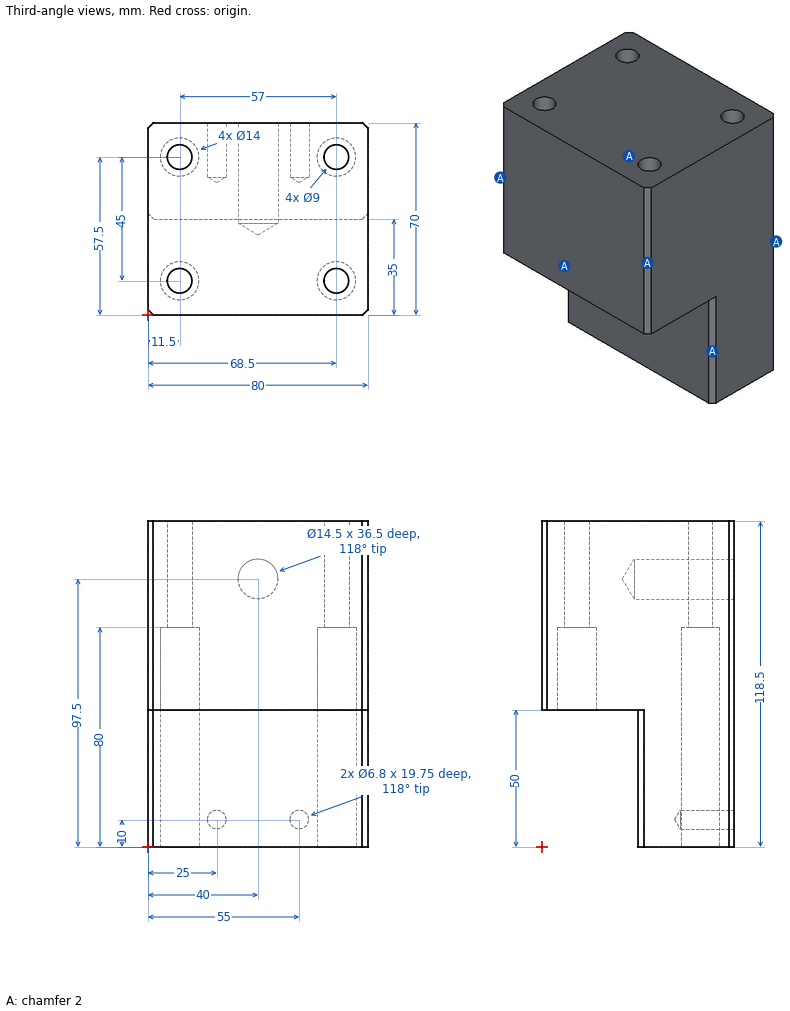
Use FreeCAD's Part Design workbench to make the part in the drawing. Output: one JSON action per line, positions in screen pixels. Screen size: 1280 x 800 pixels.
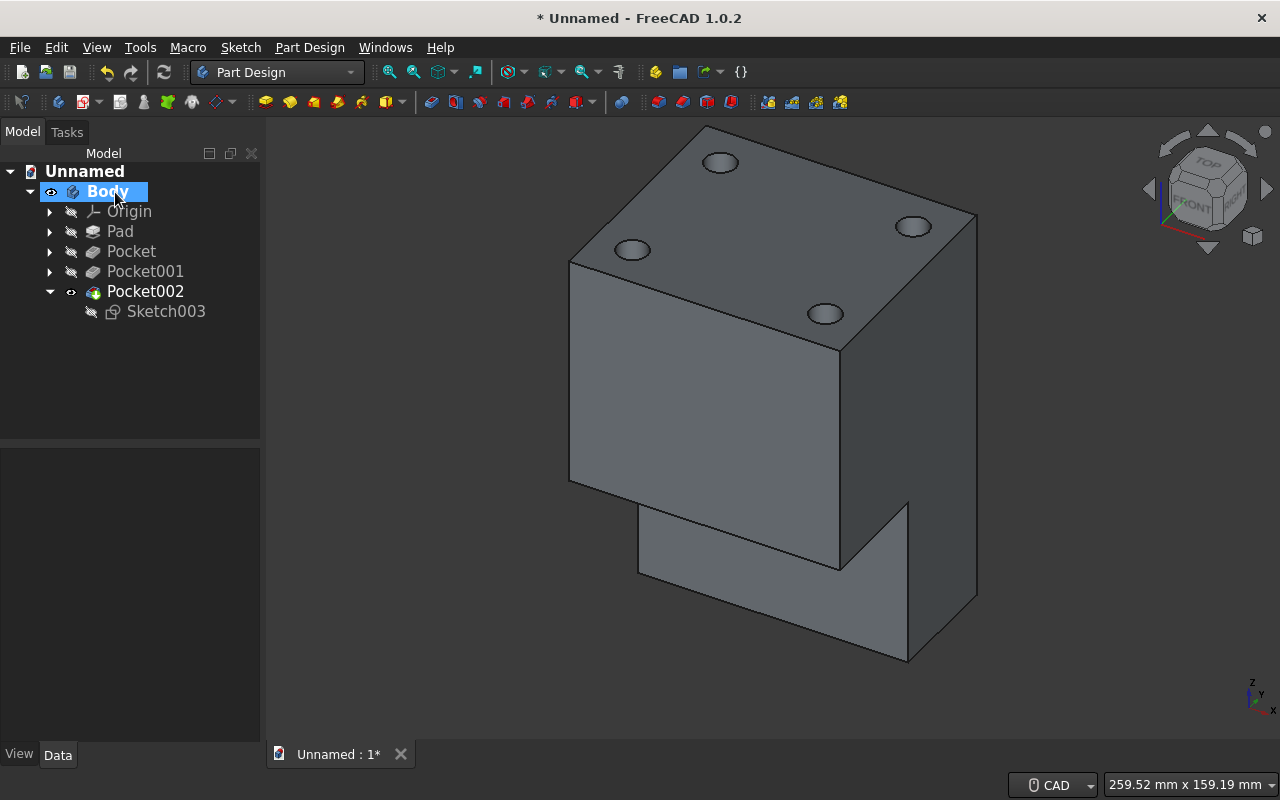
{"action": "key", "text": "4"}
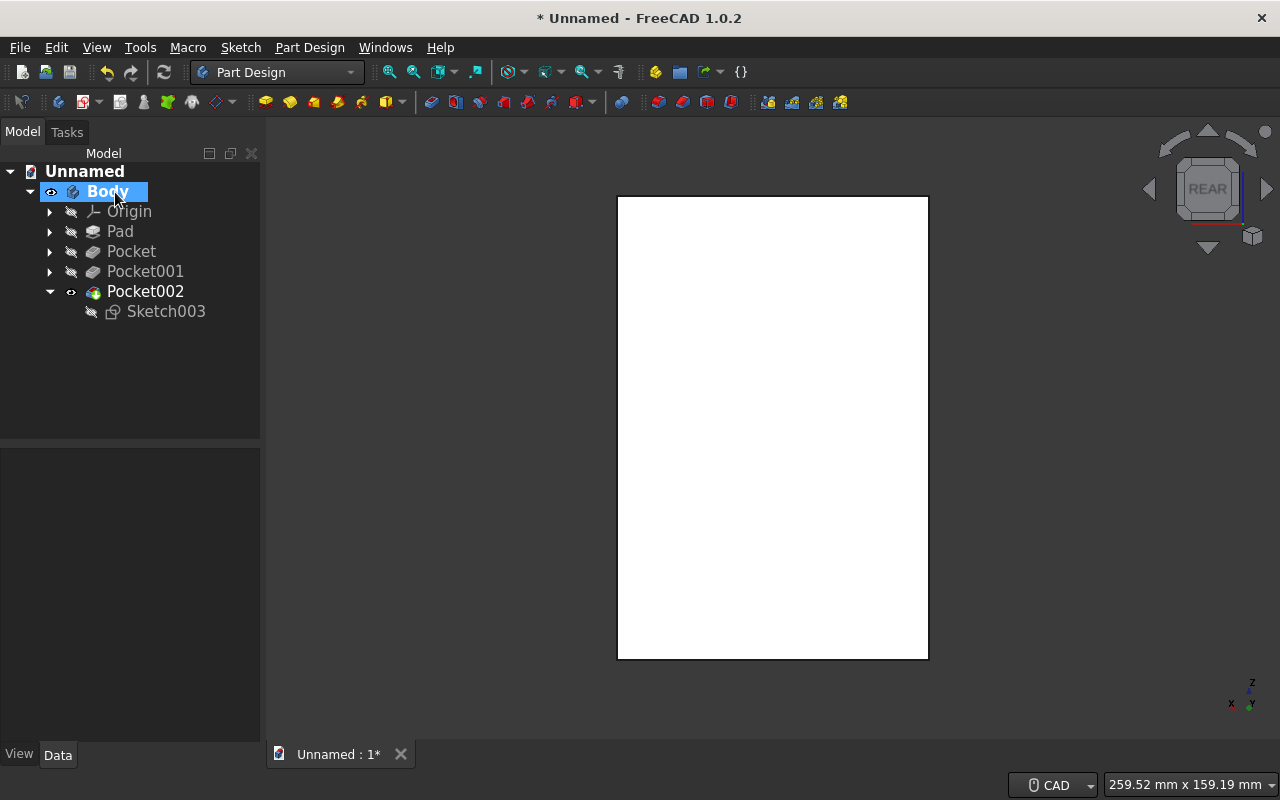
{"action": "left_click", "coordinate": [773, 361]}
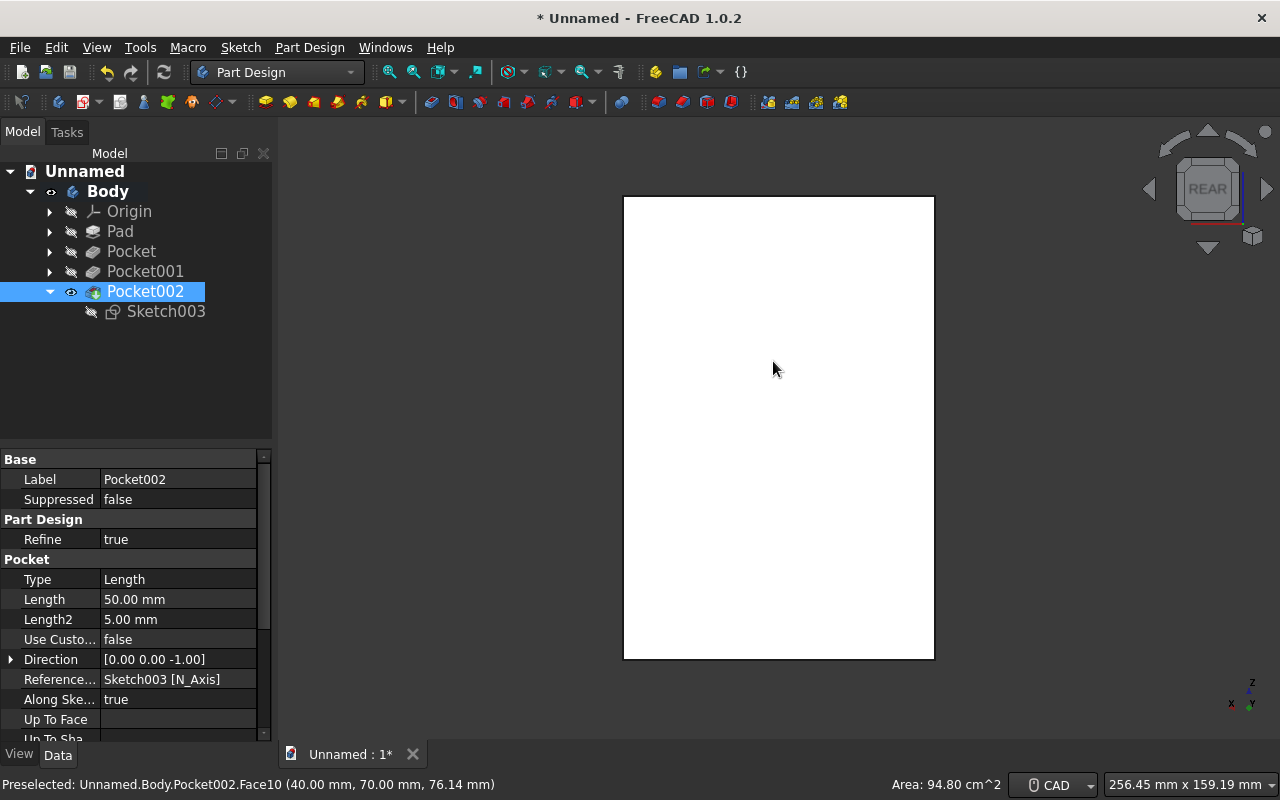
{"action": "left_click", "coordinate": [84, 102]}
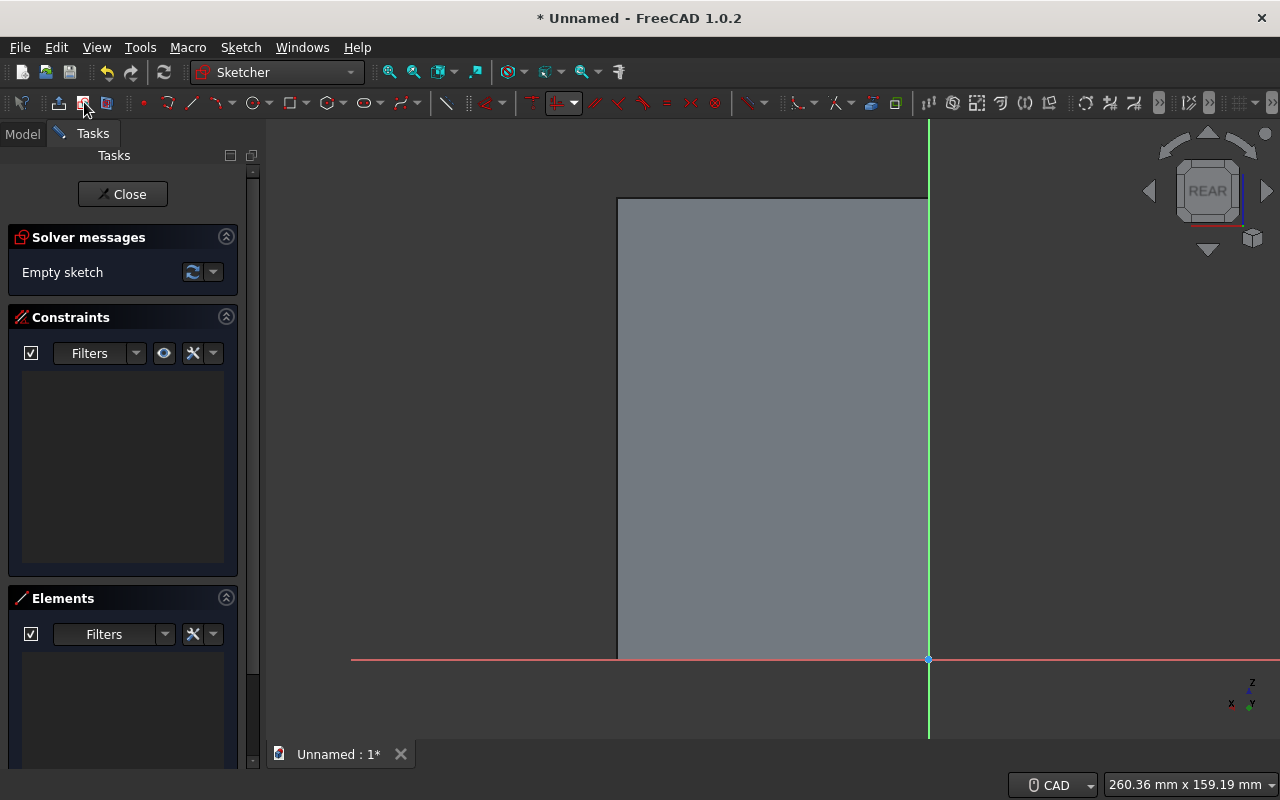
{"action": "scroll", "coordinate": [784, 257], "scroll_direction": "up", "scroll_amount": 10}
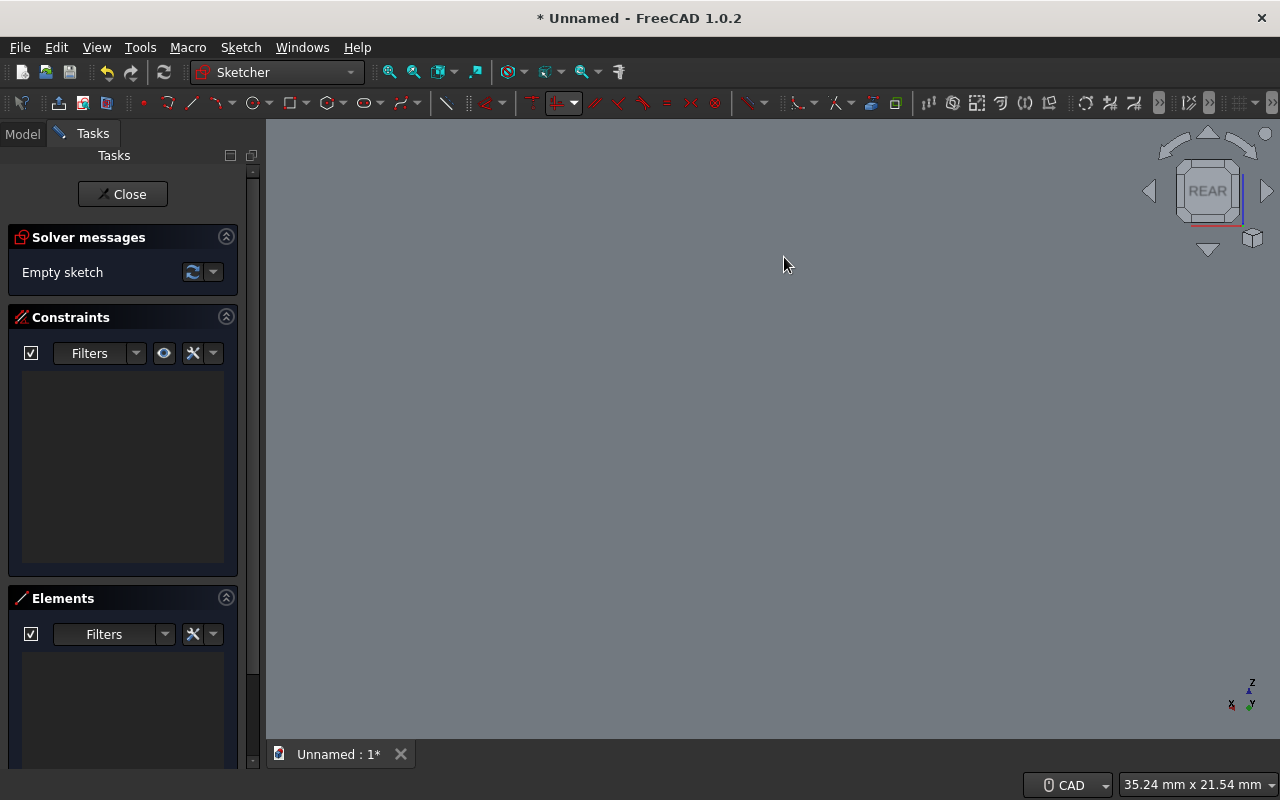
{"action": "key", "text": "g c"}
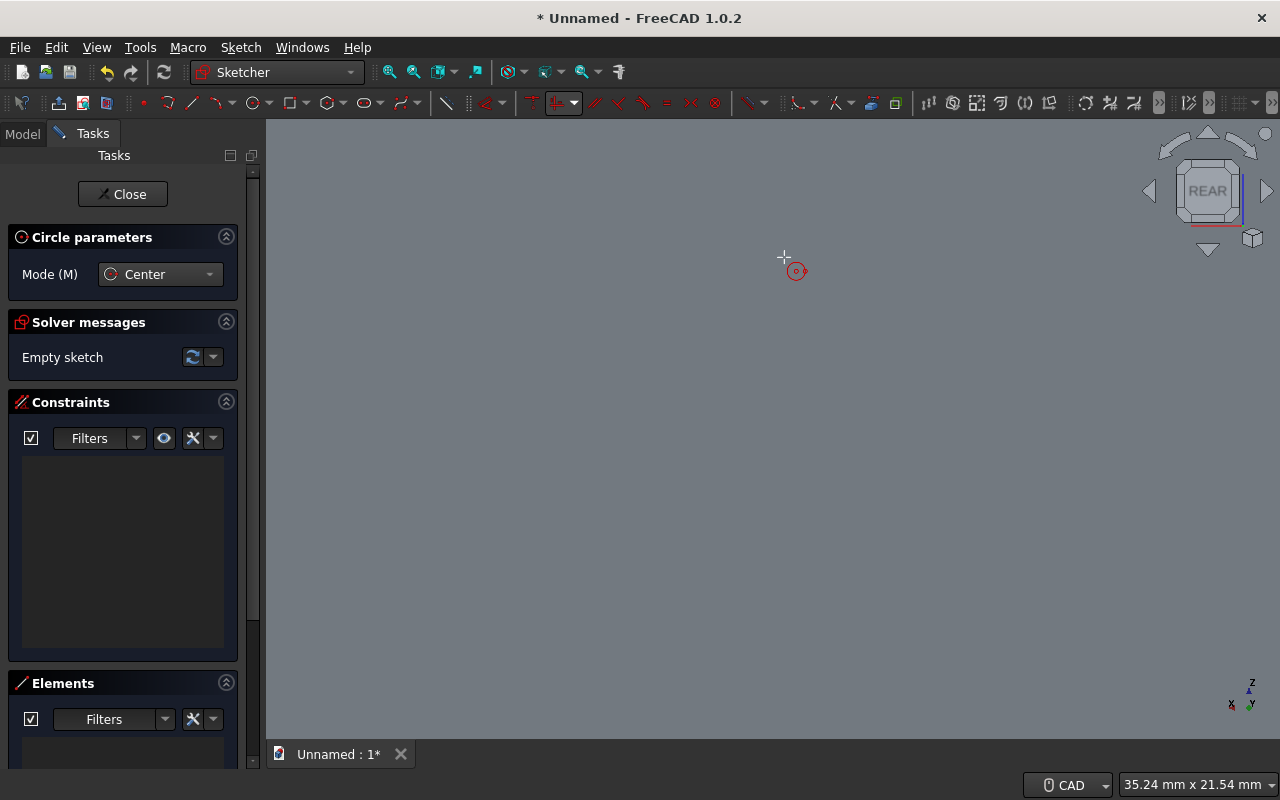
{"action": "left_click", "coordinate": [699, 426]}
{"action": "left_click", "coordinate": [847, 278]}
{"action": "key", "text": "Escape"}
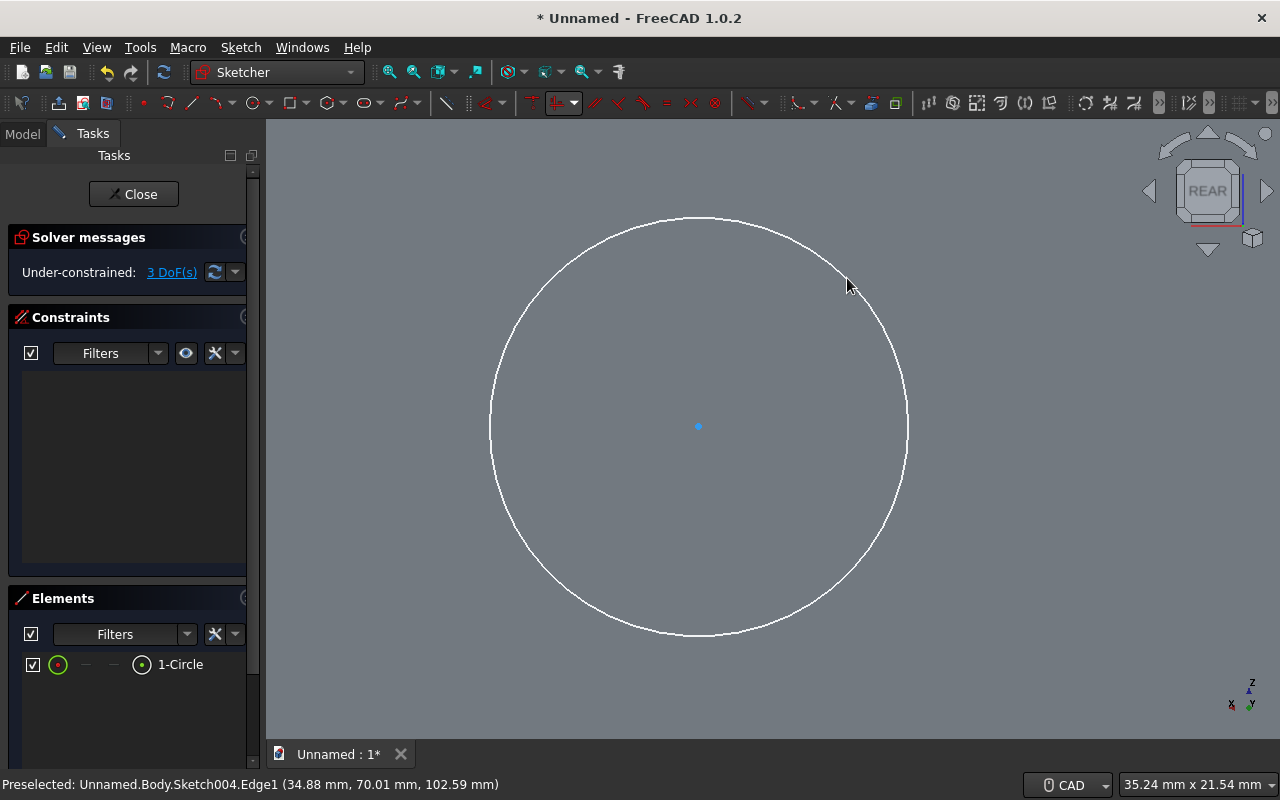
{"action": "key", "text": "d"}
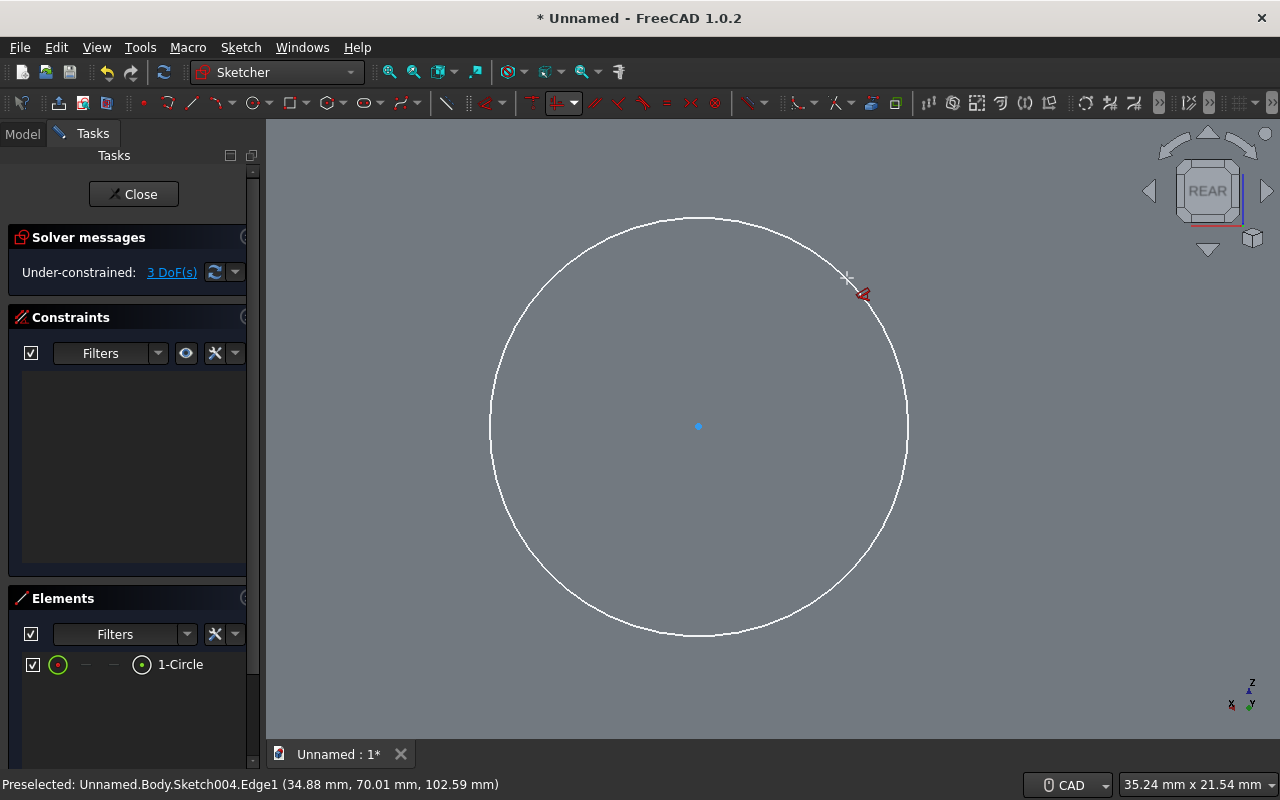
{"action": "left_click", "coordinate": [847, 279]}
{"action": "left_click", "coordinate": [870, 256]}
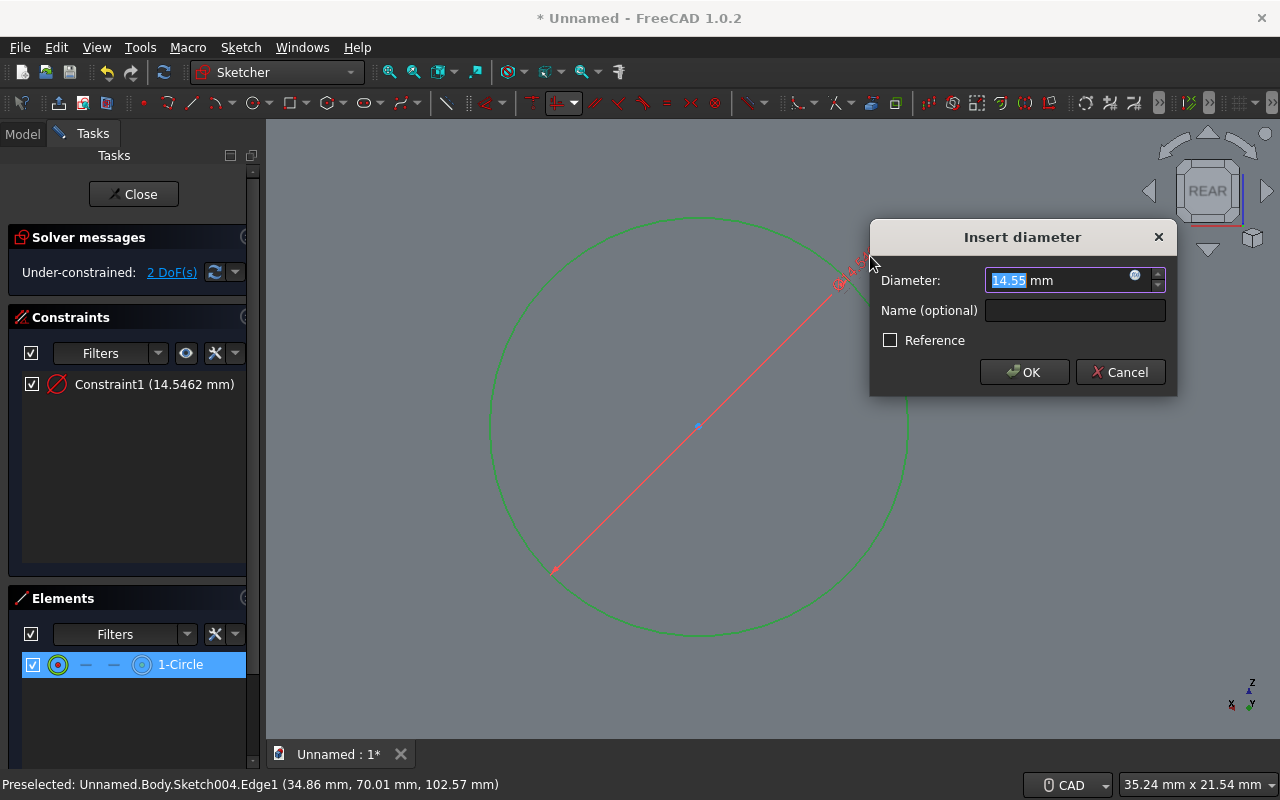
{"action": "type", "text": "14.5"}
{"action": "key", "text": "Return"}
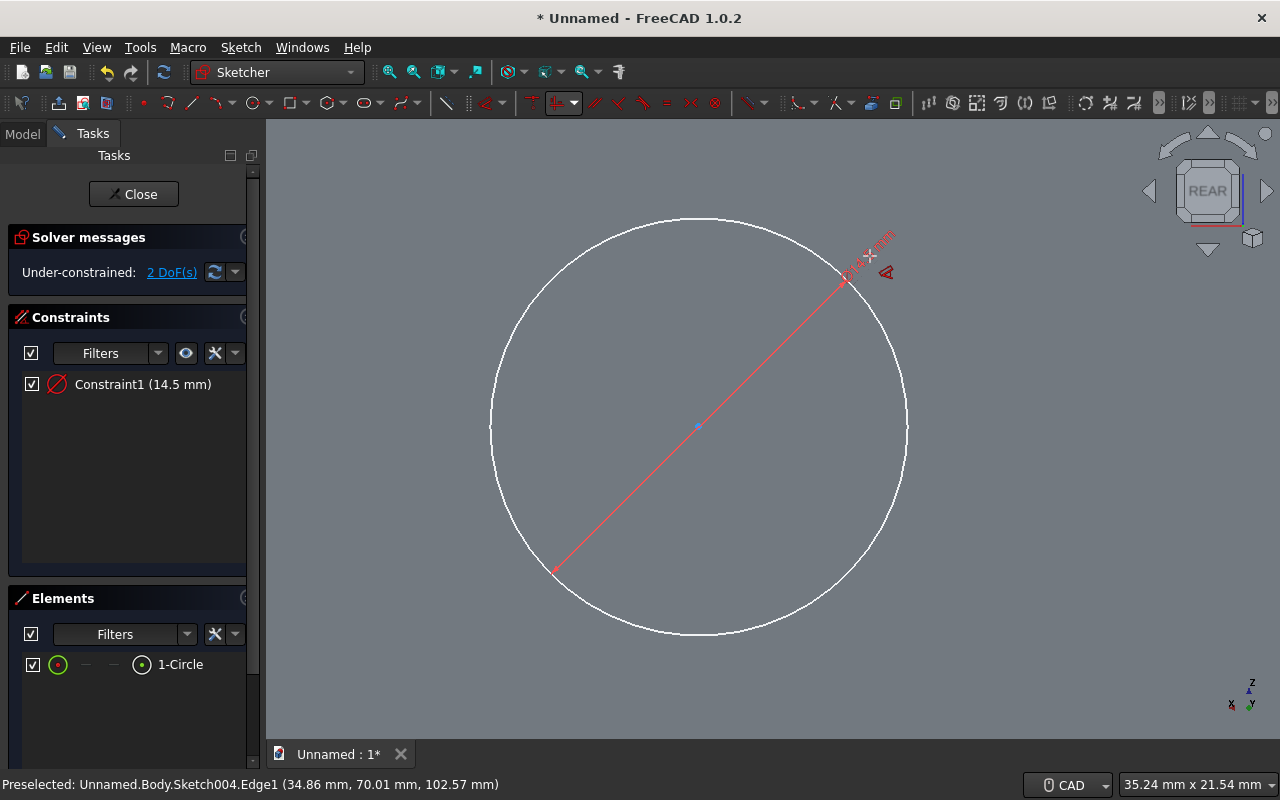
{"action": "left_click", "coordinate": [699, 427]}
{"action": "left_click", "coordinate": [811, 393]}